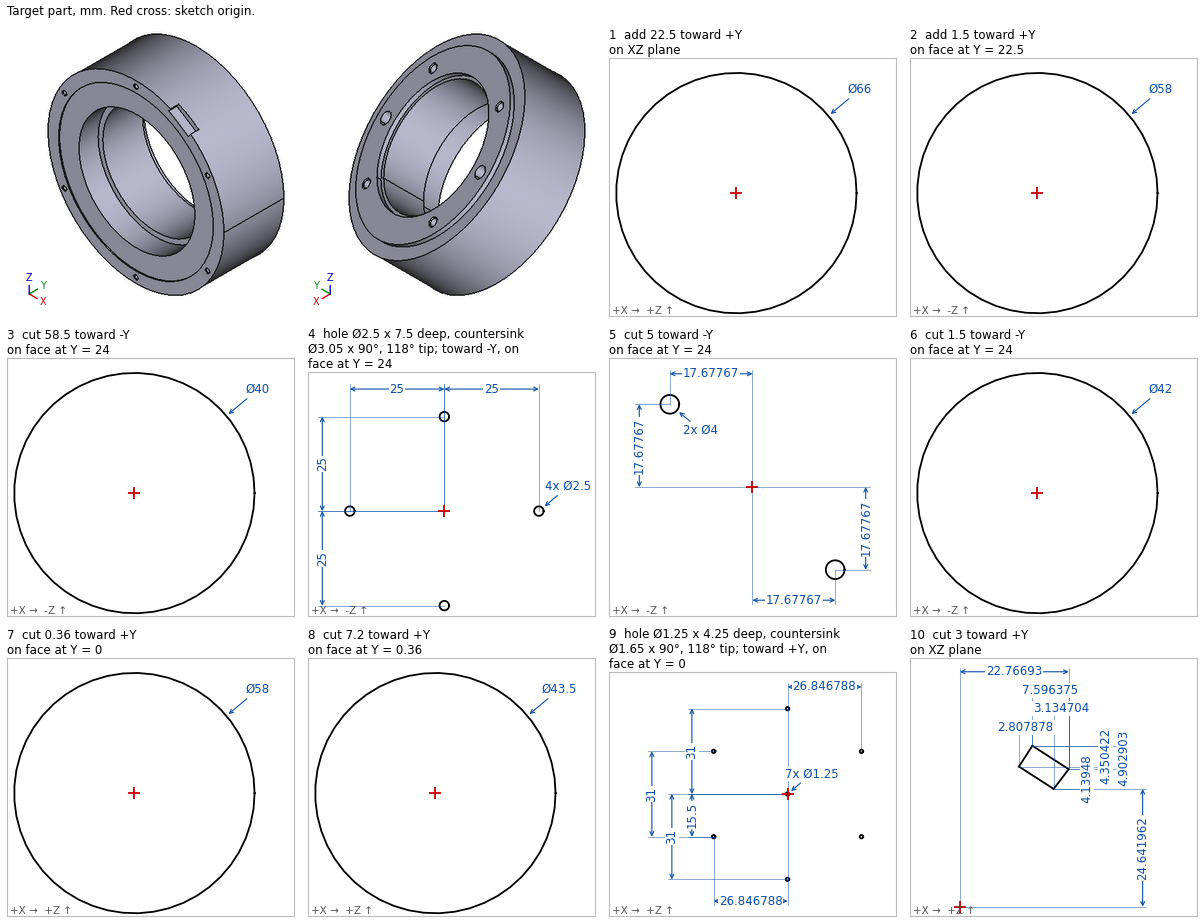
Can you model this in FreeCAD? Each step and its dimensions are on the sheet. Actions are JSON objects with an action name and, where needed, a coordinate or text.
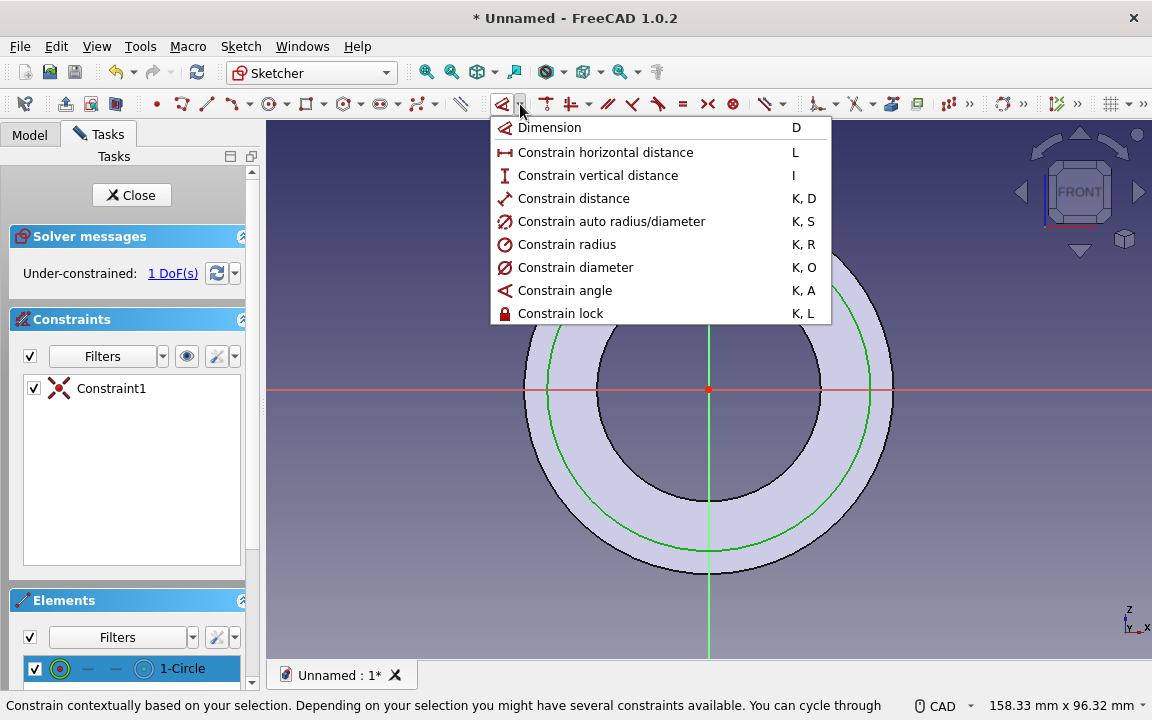
{"action": "left_click", "coordinate": [661, 268]}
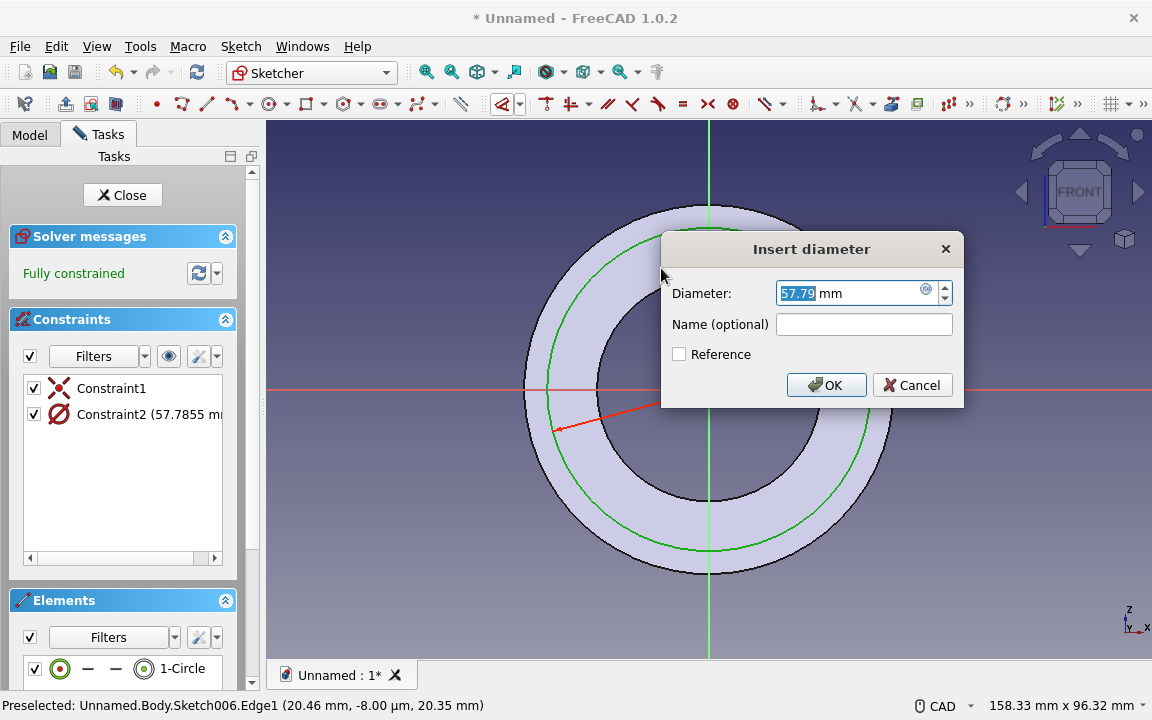
{"action": "type", "text": "58"}
{"action": "key", "text": "Return"}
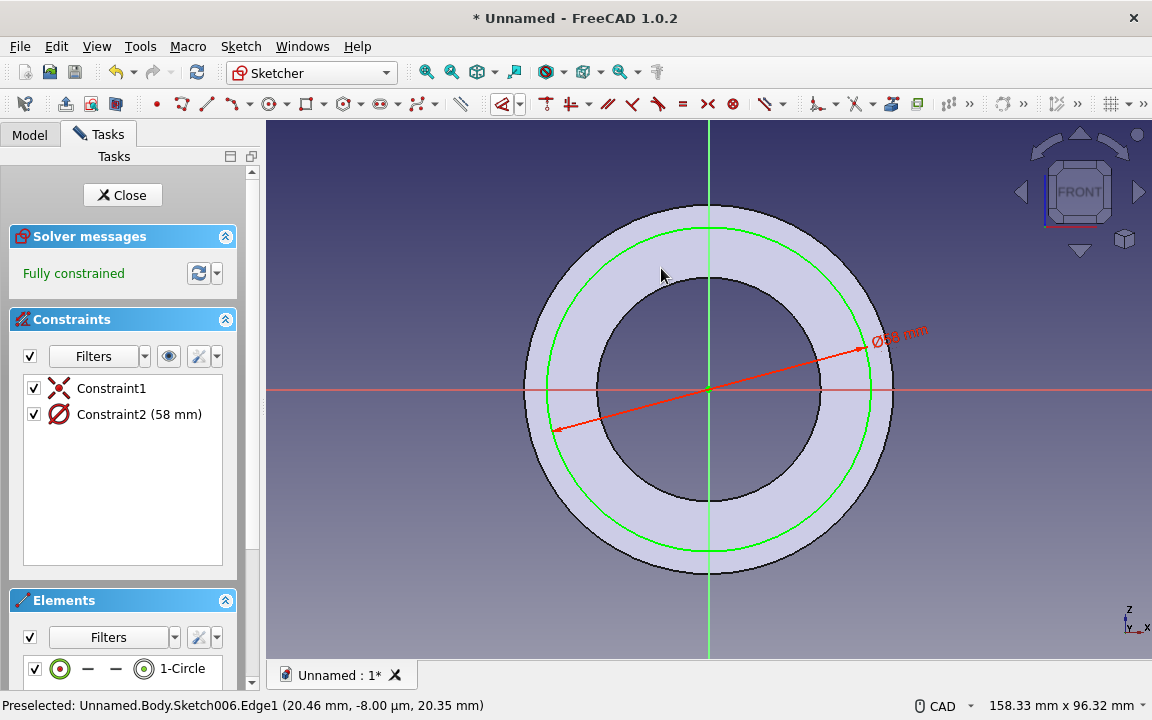
{"action": "left_click", "coordinate": [123, 195]}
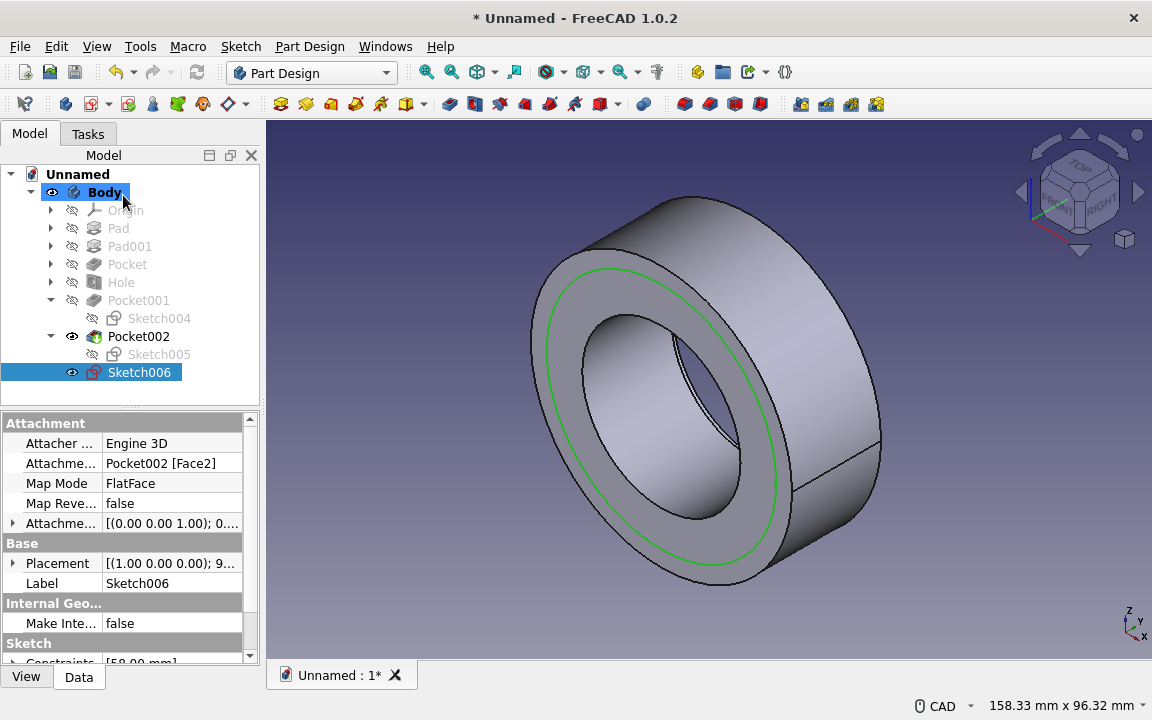
{"action": "left_click", "coordinate": [450, 104]}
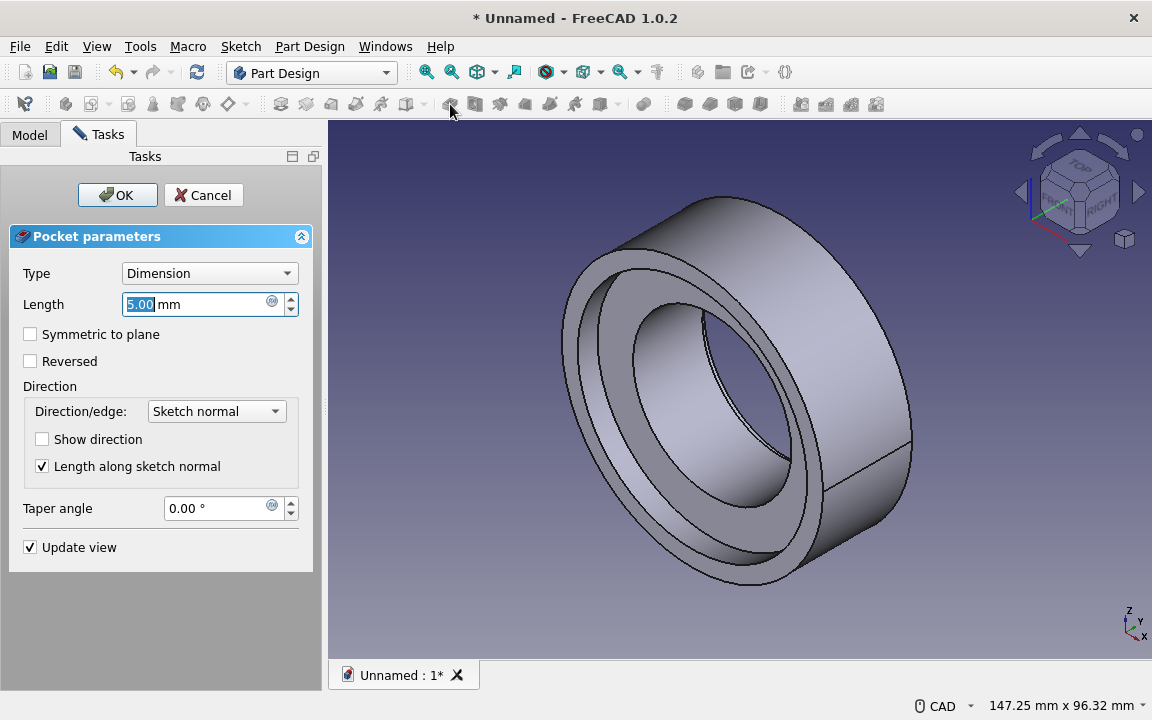
{"action": "type", "text": "0.36"}
{"action": "key", "text": "Tab"}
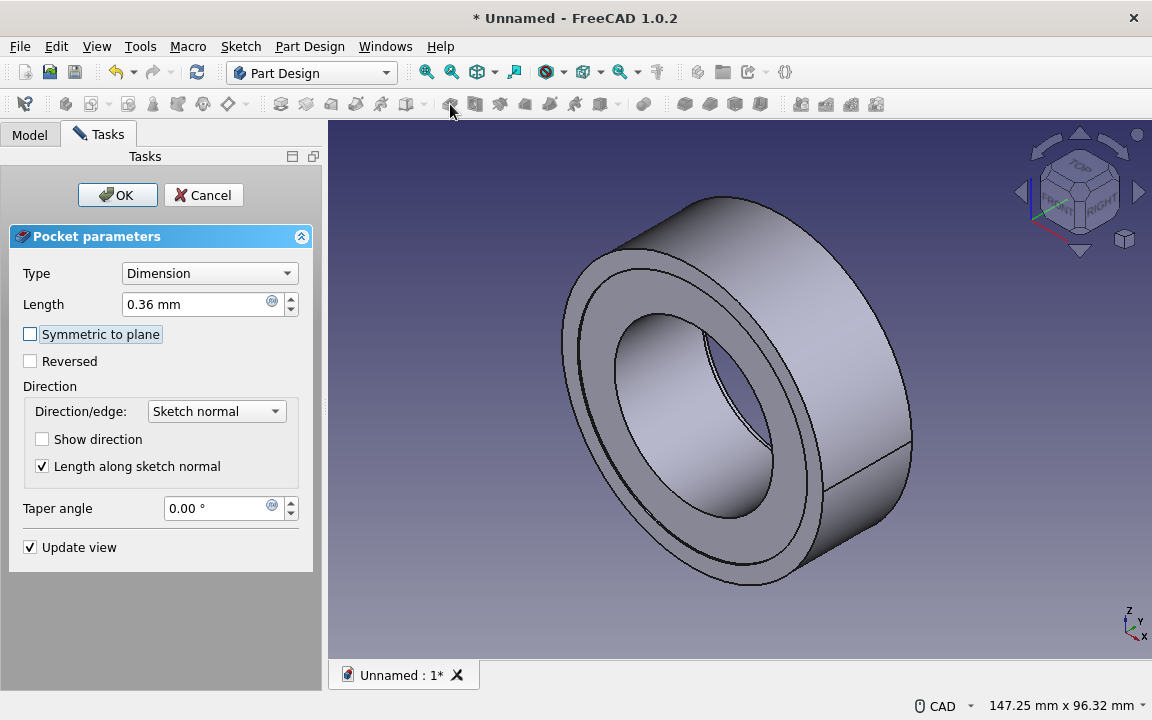
{"action": "left_click", "coordinate": [118, 195]}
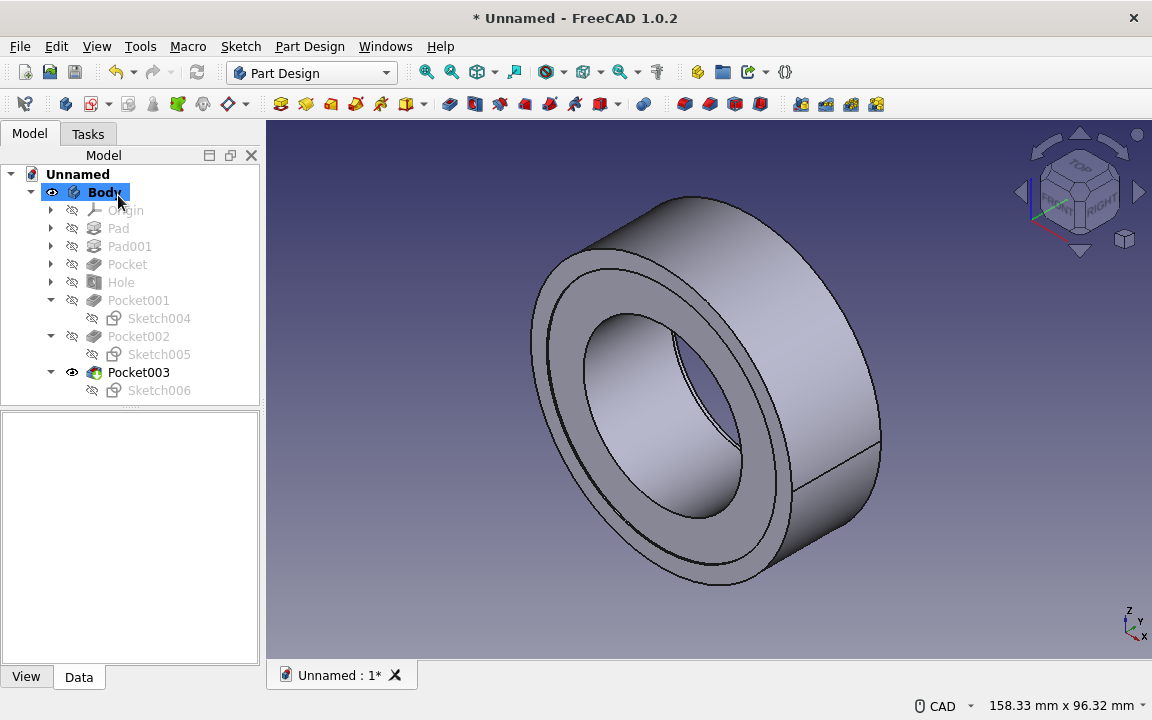
{"action": "left_click", "coordinate": [761, 472]}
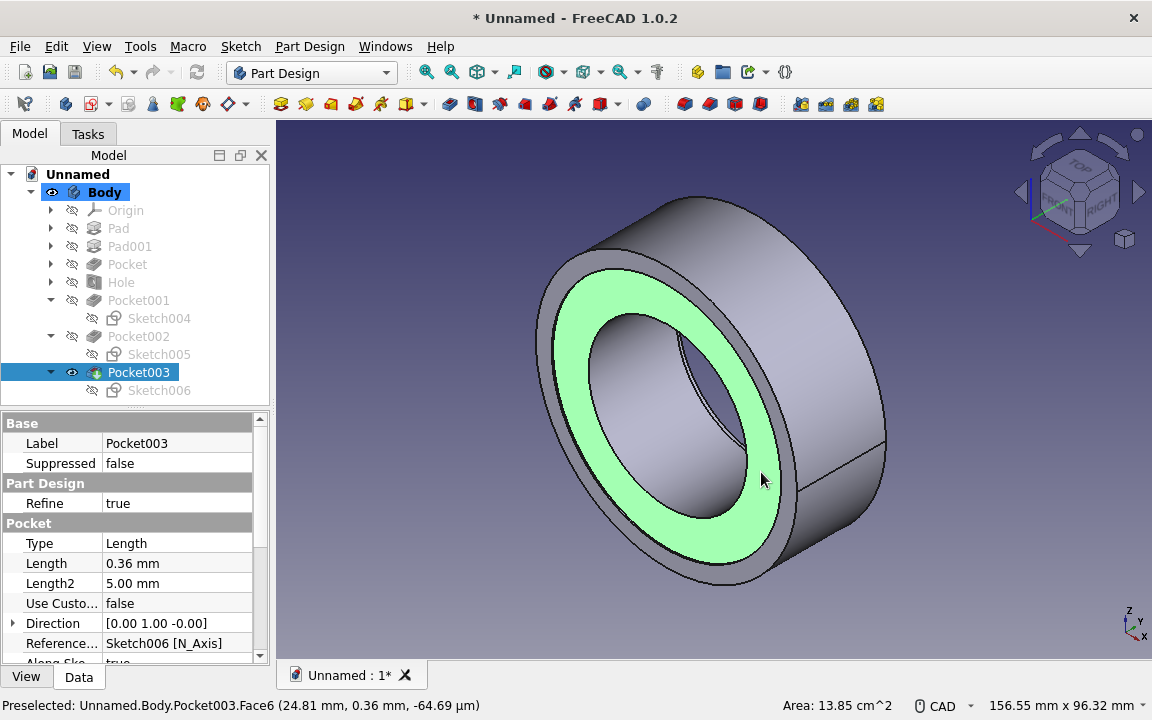
{"action": "left_click", "coordinate": [90, 104]}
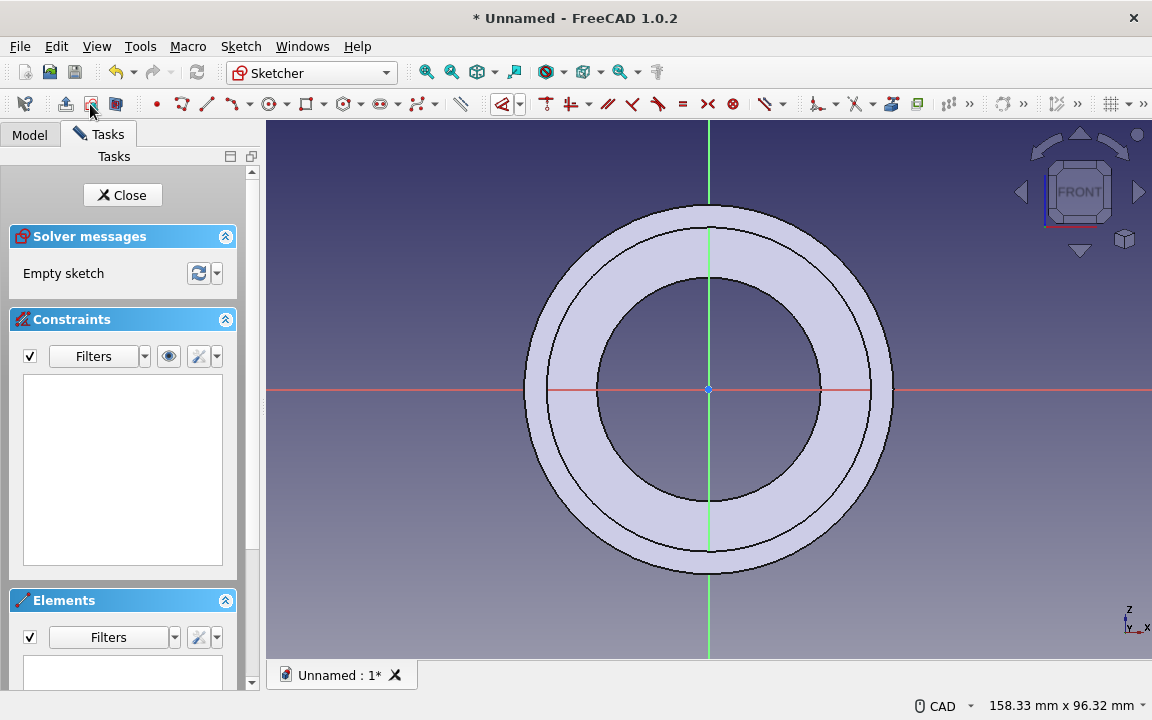
{"action": "left_click", "coordinate": [116, 104]}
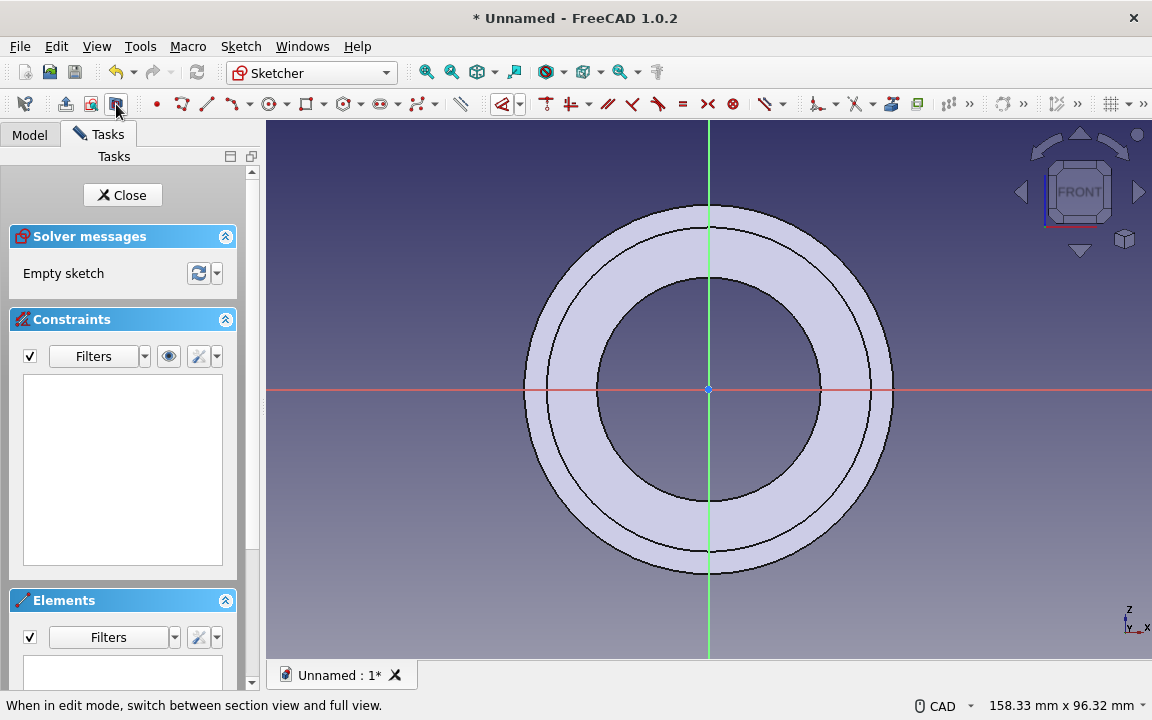
{"action": "scroll", "coordinate": [848, 390], "scroll_direction": "up", "scroll_amount": 2}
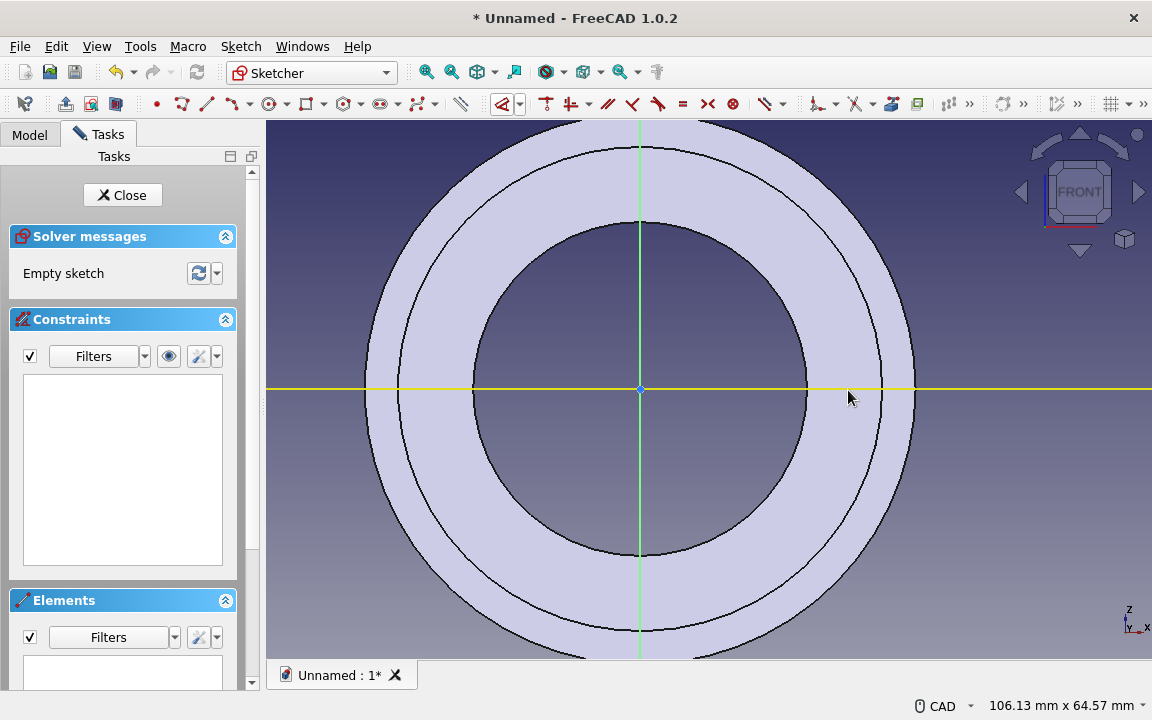
{"action": "left_click", "coordinate": [268, 104]}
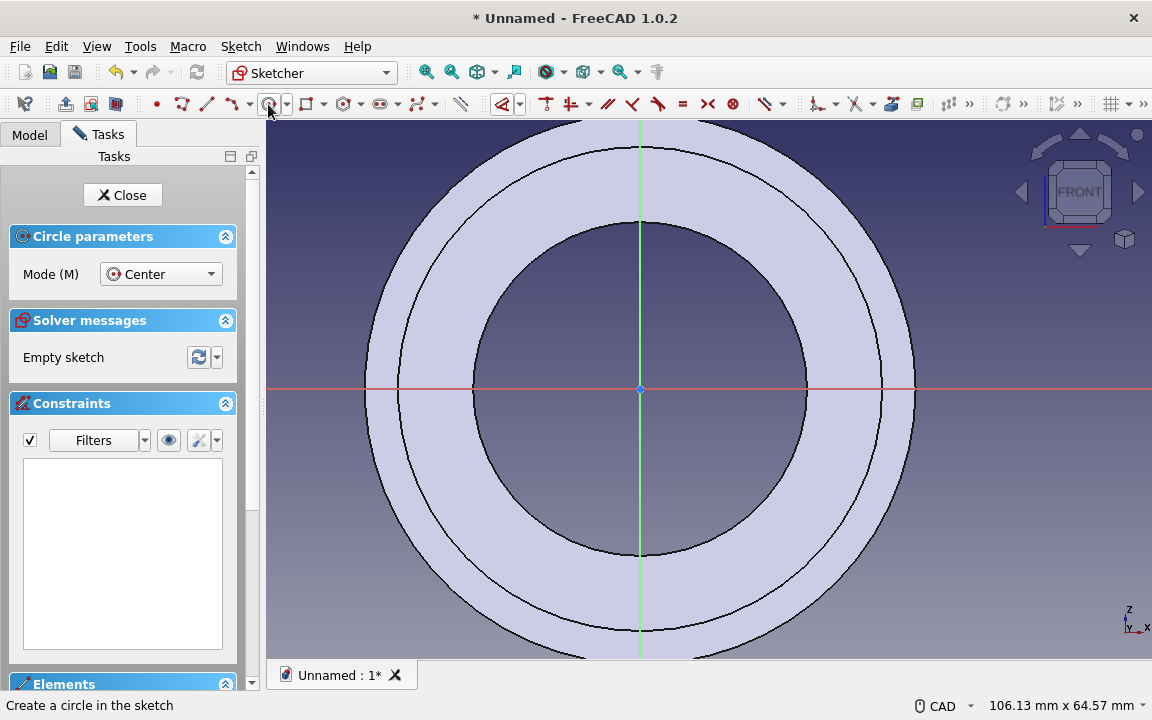
{"action": "left_click", "coordinate": [640, 389]}
{"action": "left_click", "coordinate": [768, 261]}
{"action": "key", "text": "Escape"}